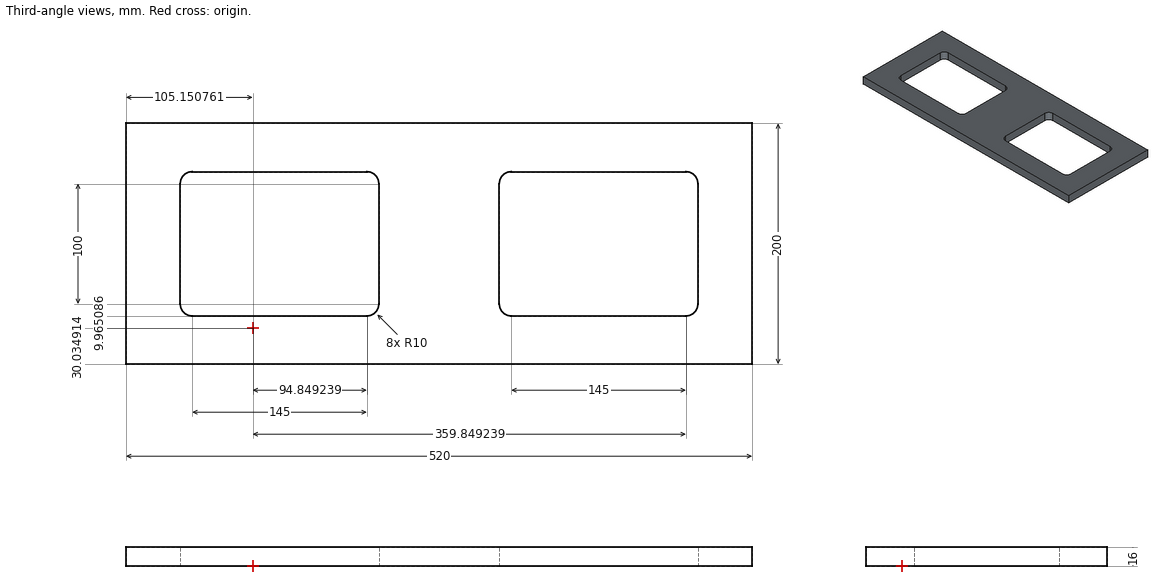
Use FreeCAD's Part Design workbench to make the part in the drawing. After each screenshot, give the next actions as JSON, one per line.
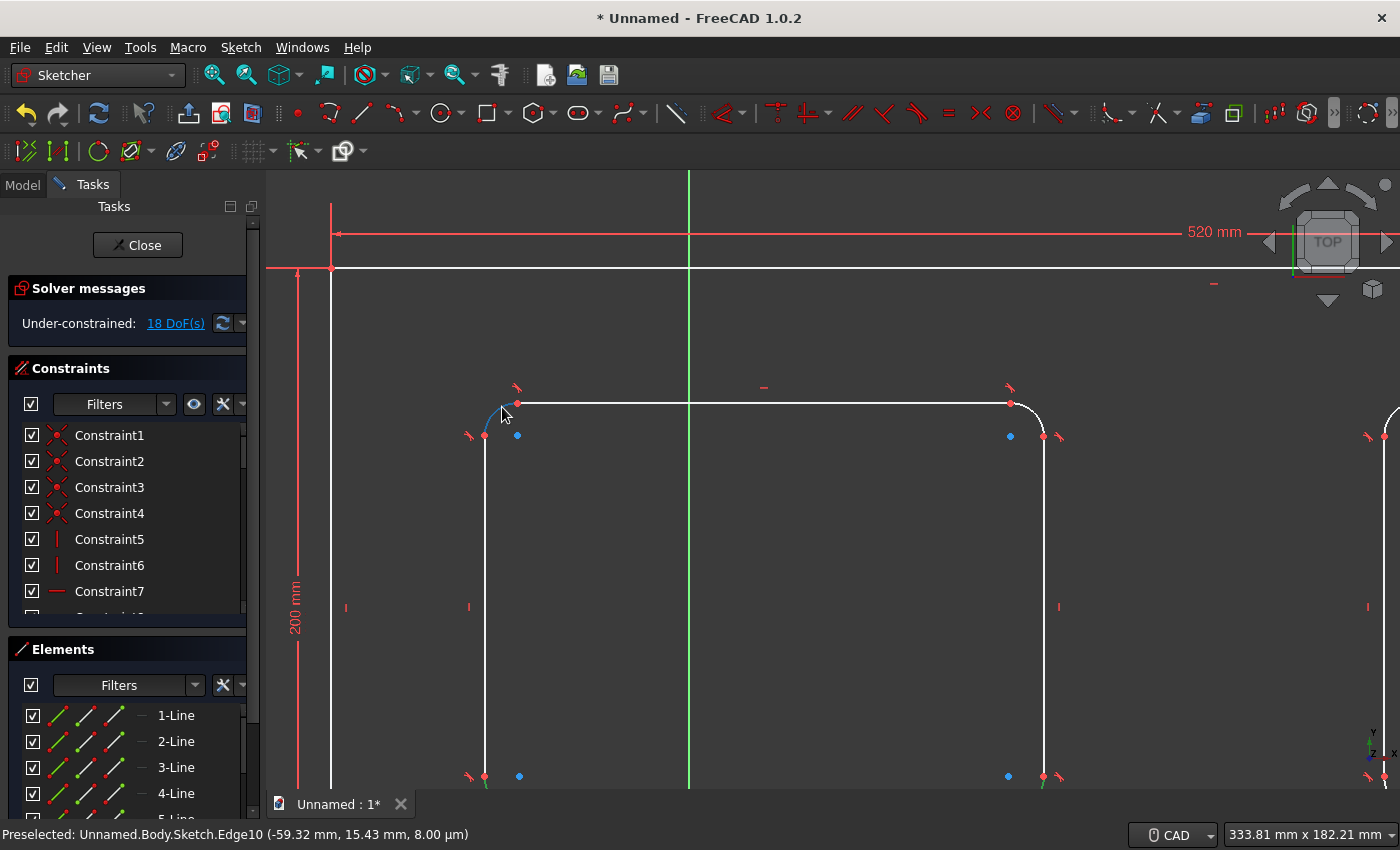
{"action": "left_click", "coordinate": [503, 407]}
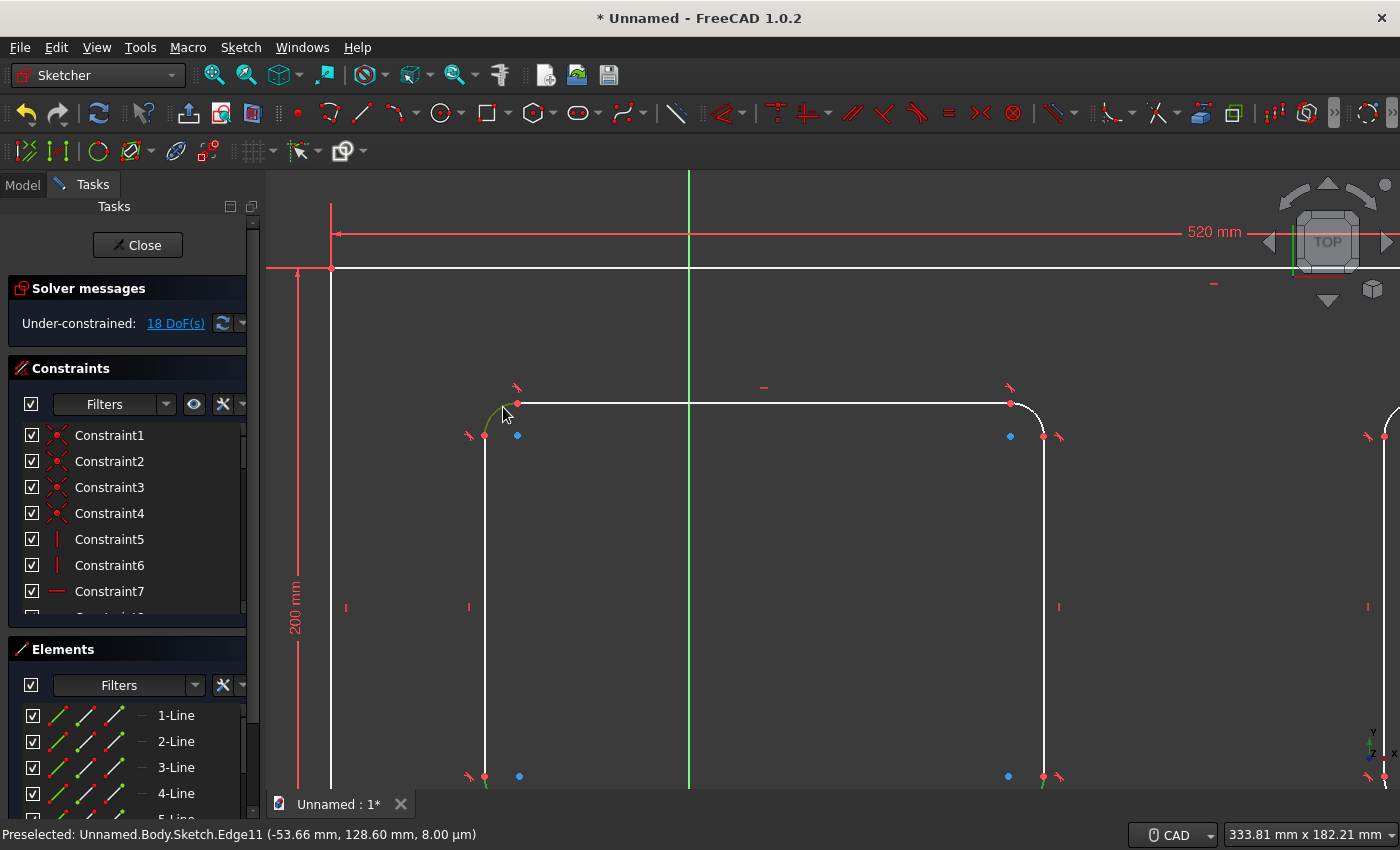
{"action": "left_click", "coordinate": [1040, 421]}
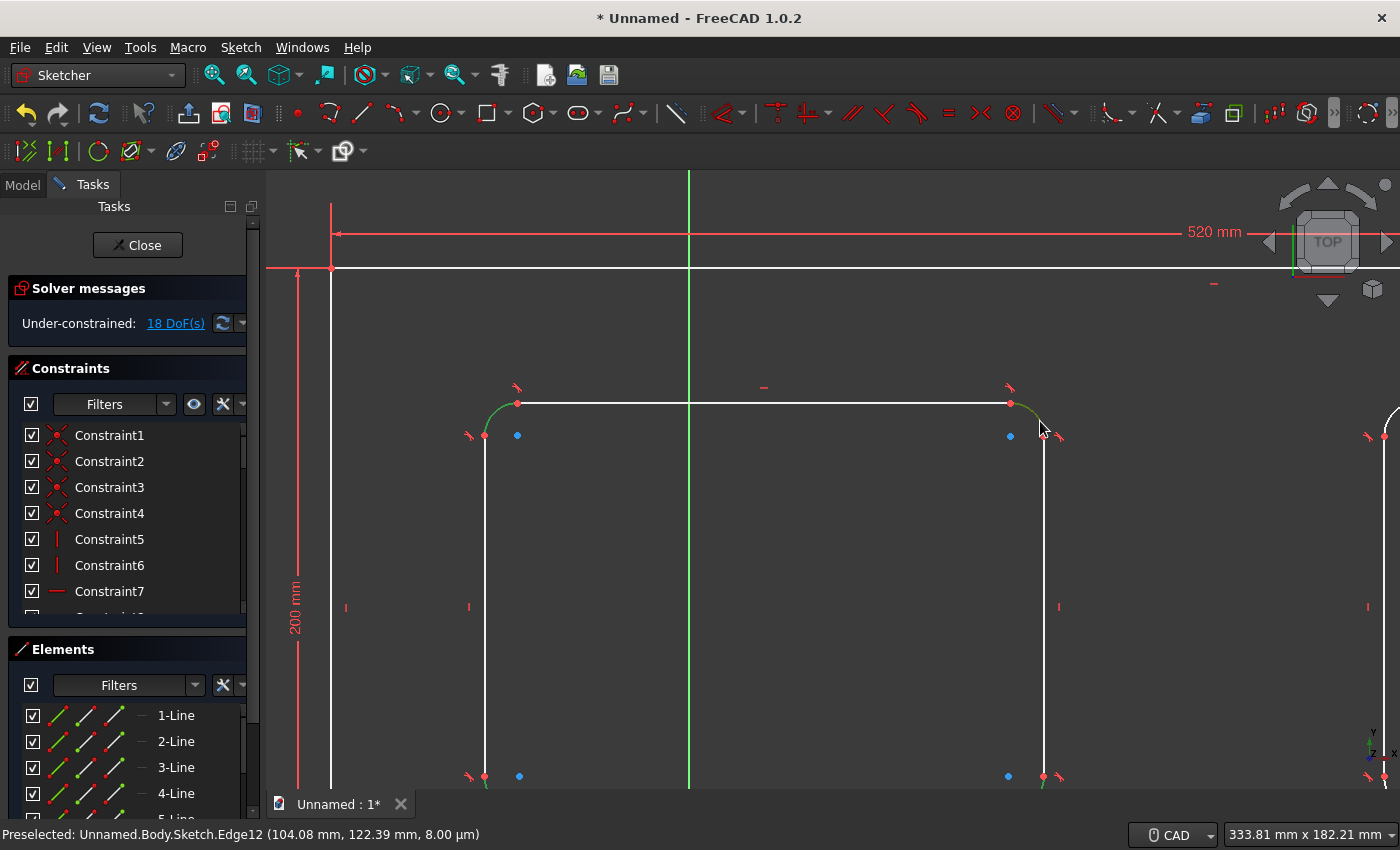
{"action": "scroll", "coordinate": [502, 407], "scroll_direction": "down", "scroll_amount": 5}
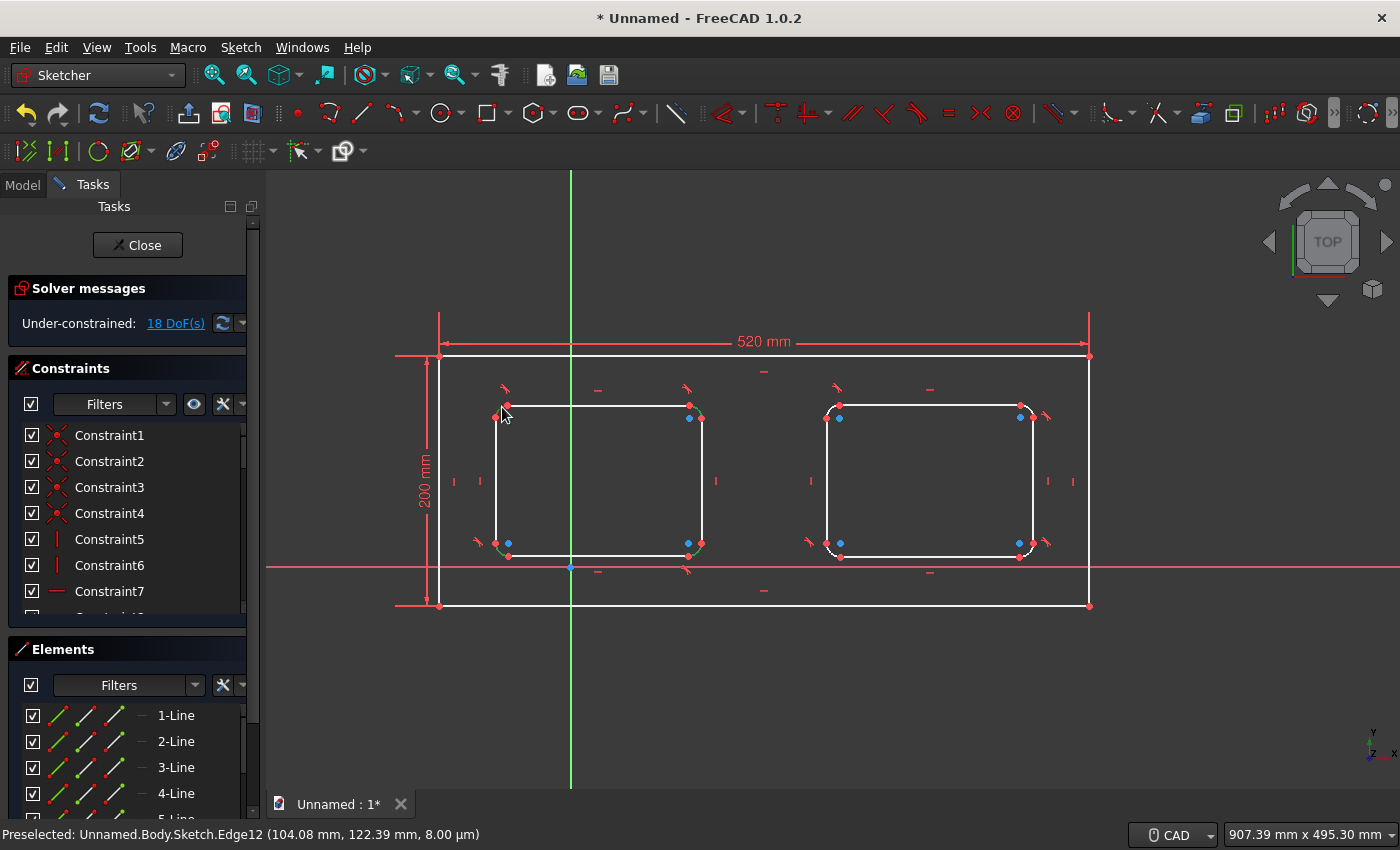
{"action": "scroll", "coordinate": [828, 549], "scroll_direction": "up", "scroll_amount": 4}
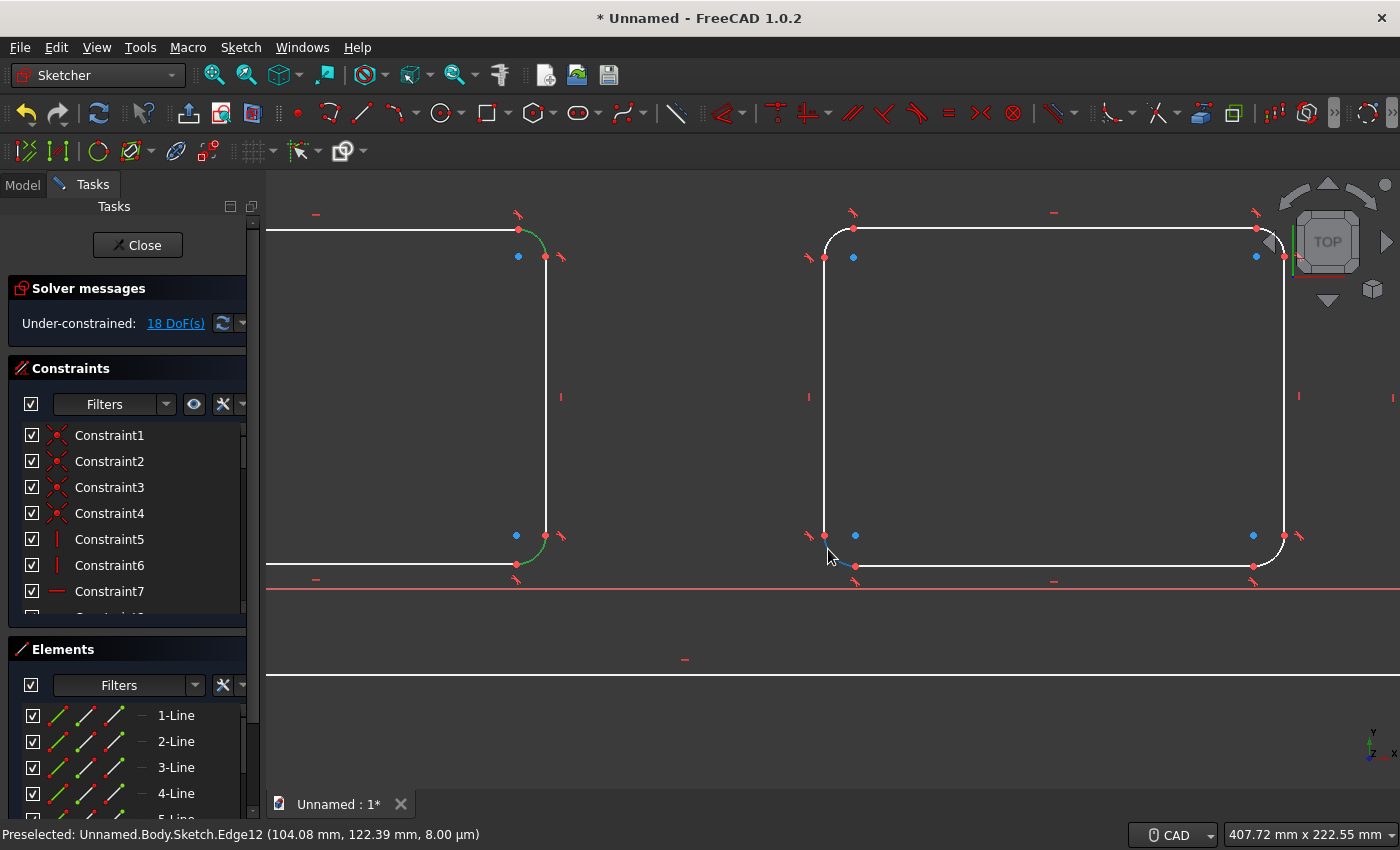
{"action": "left_click", "coordinate": [828, 549]}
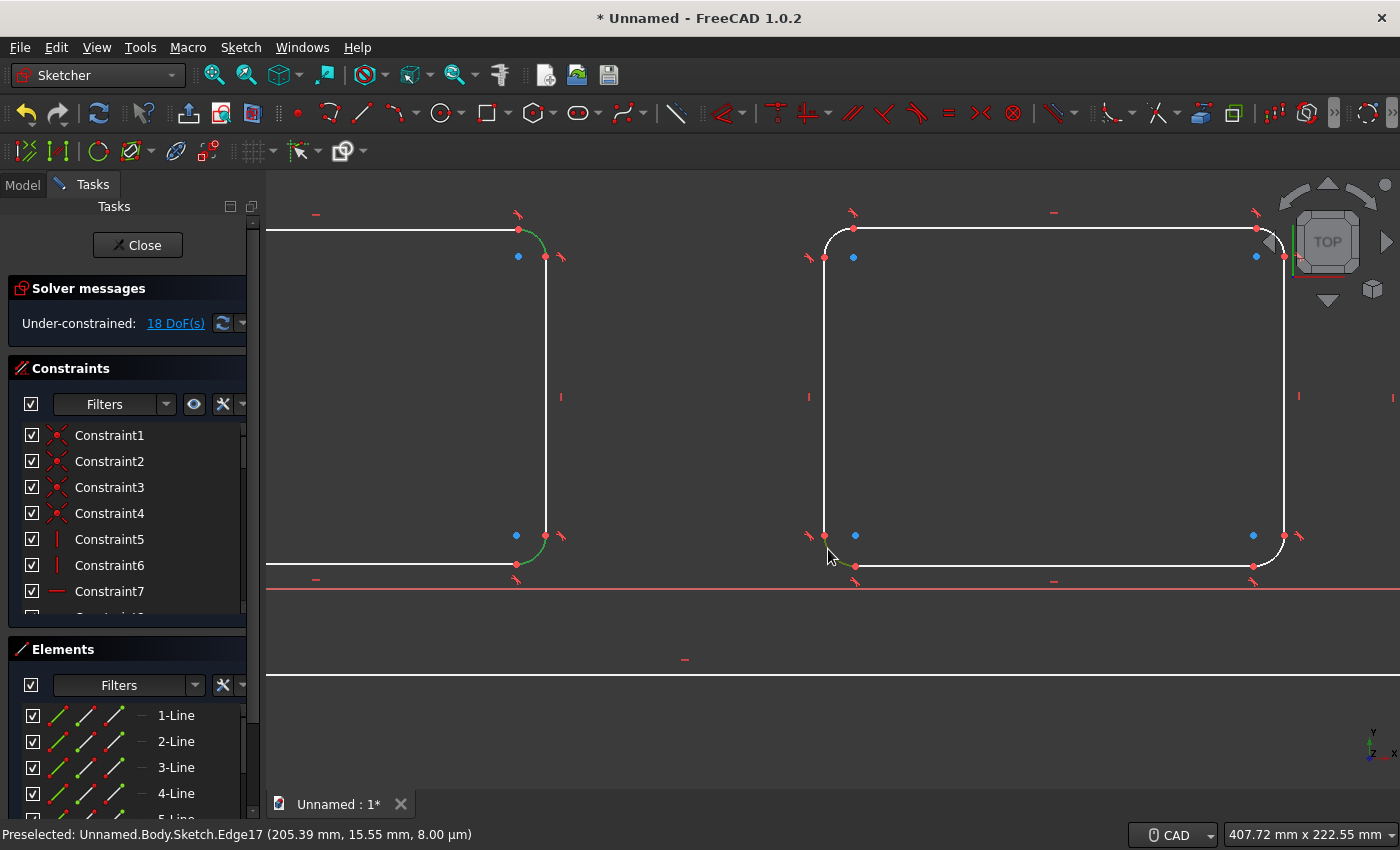
{"action": "left_click", "coordinate": [840, 231]}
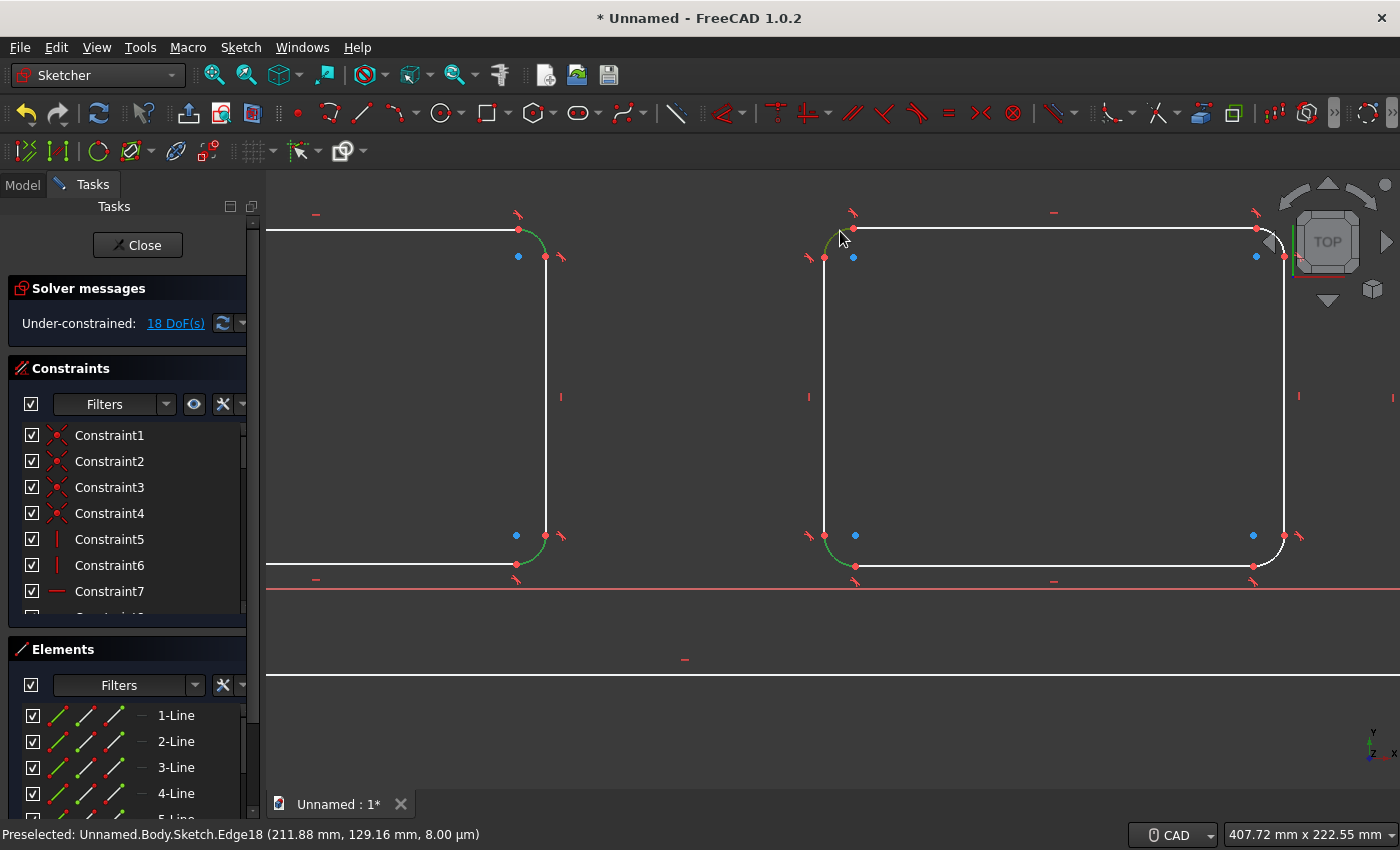
{"action": "scroll", "coordinate": [829, 549], "scroll_direction": "down", "scroll_amount": 4}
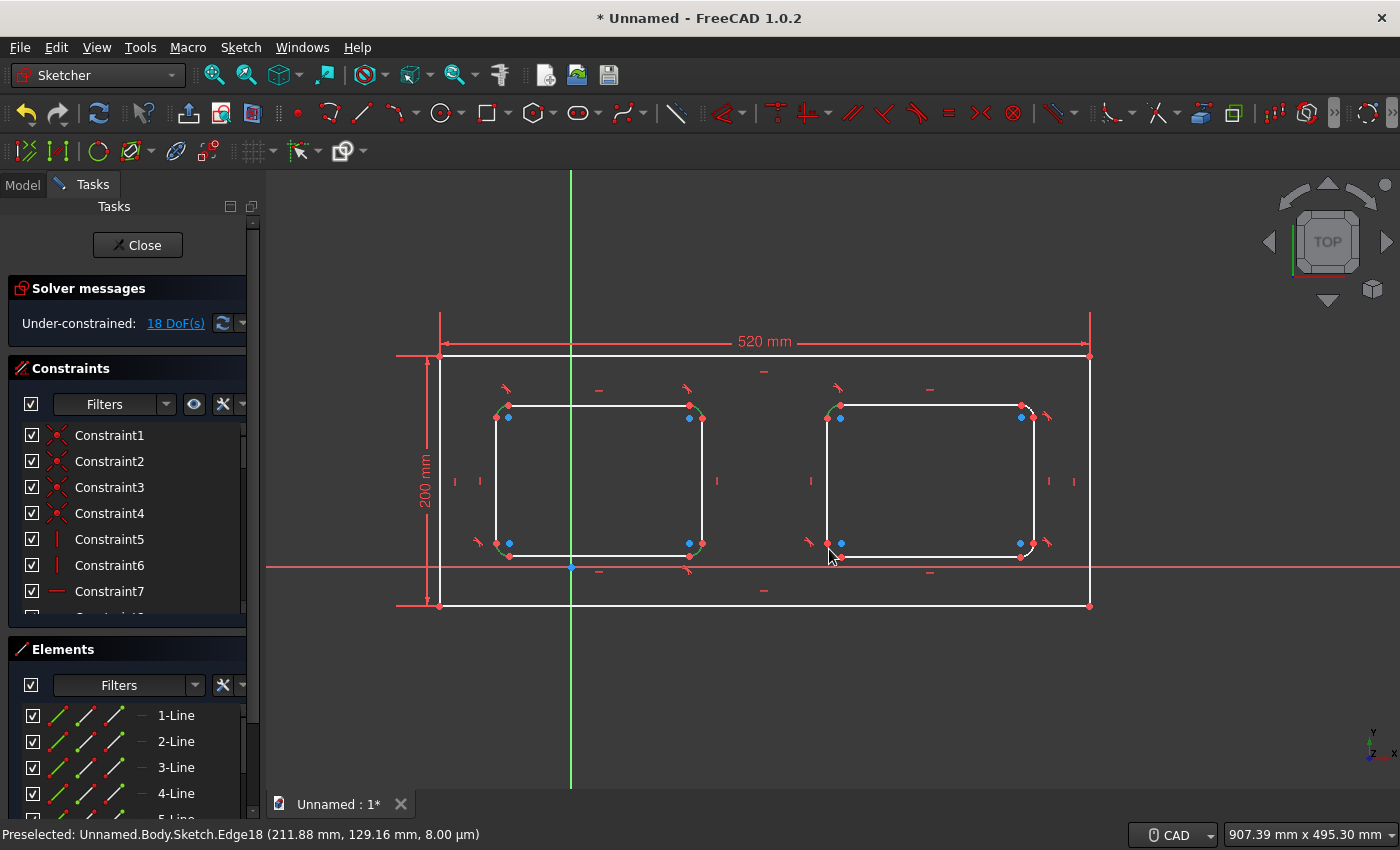
{"action": "scroll", "coordinate": [1032, 412], "scroll_direction": "up", "scroll_amount": 5}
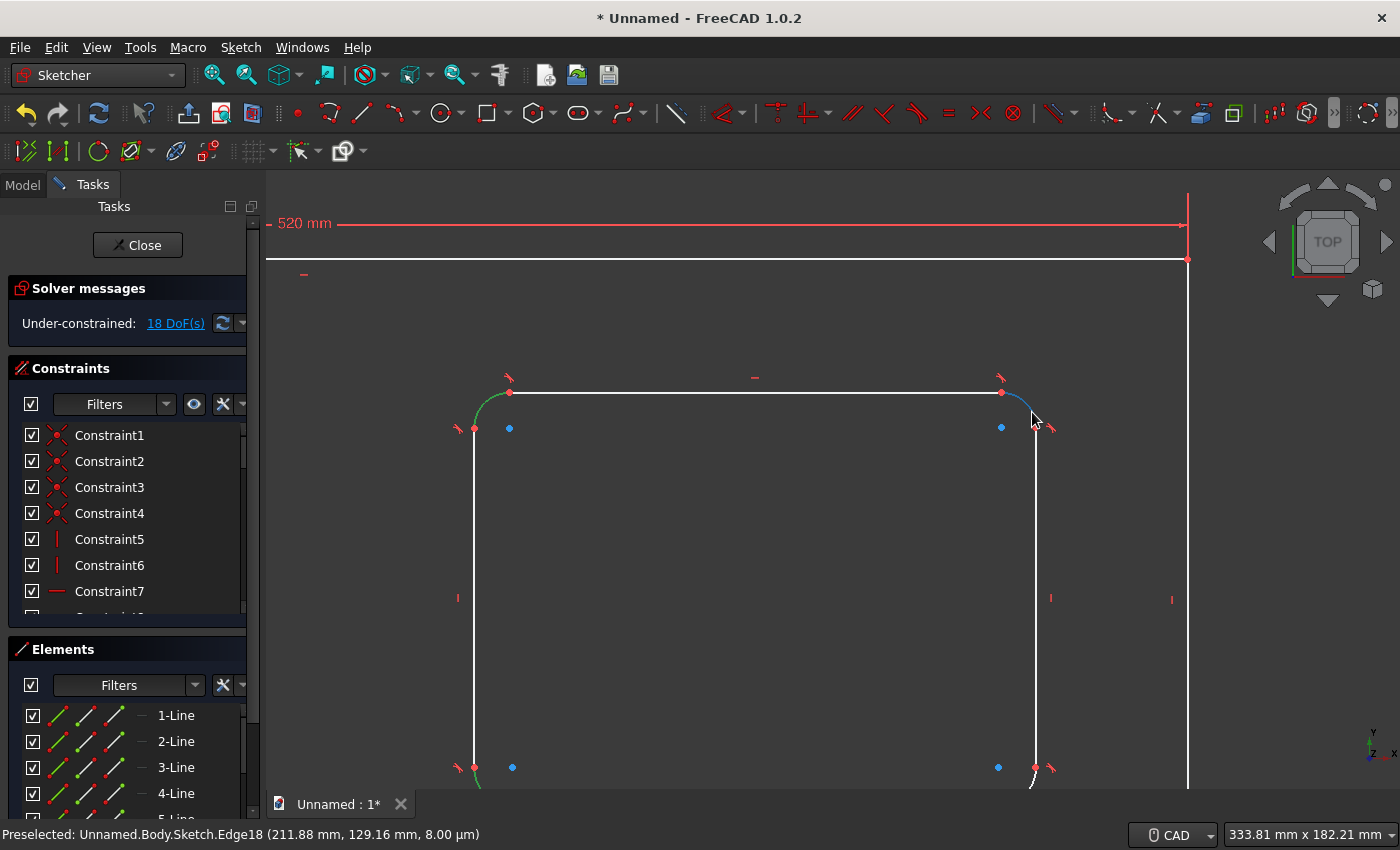
{"action": "left_click", "coordinate": [1032, 412]}